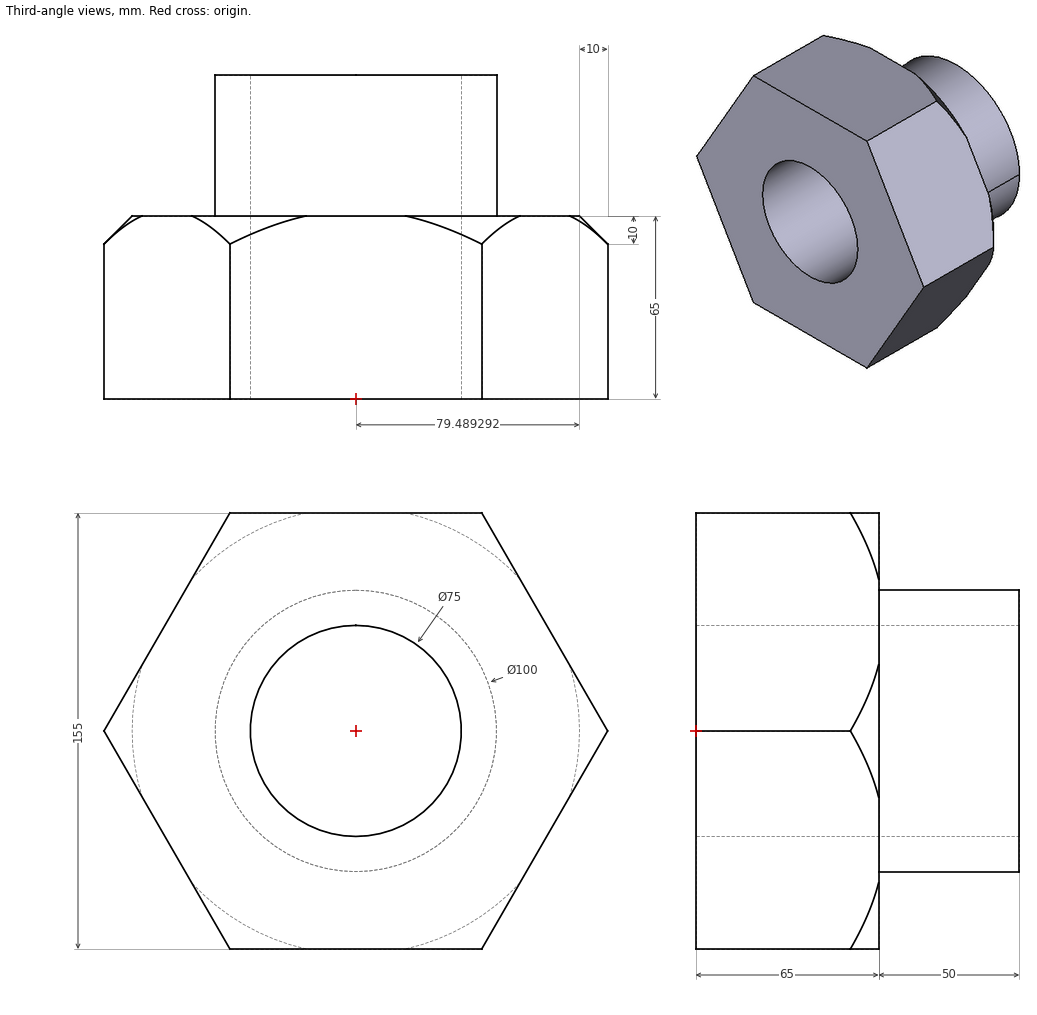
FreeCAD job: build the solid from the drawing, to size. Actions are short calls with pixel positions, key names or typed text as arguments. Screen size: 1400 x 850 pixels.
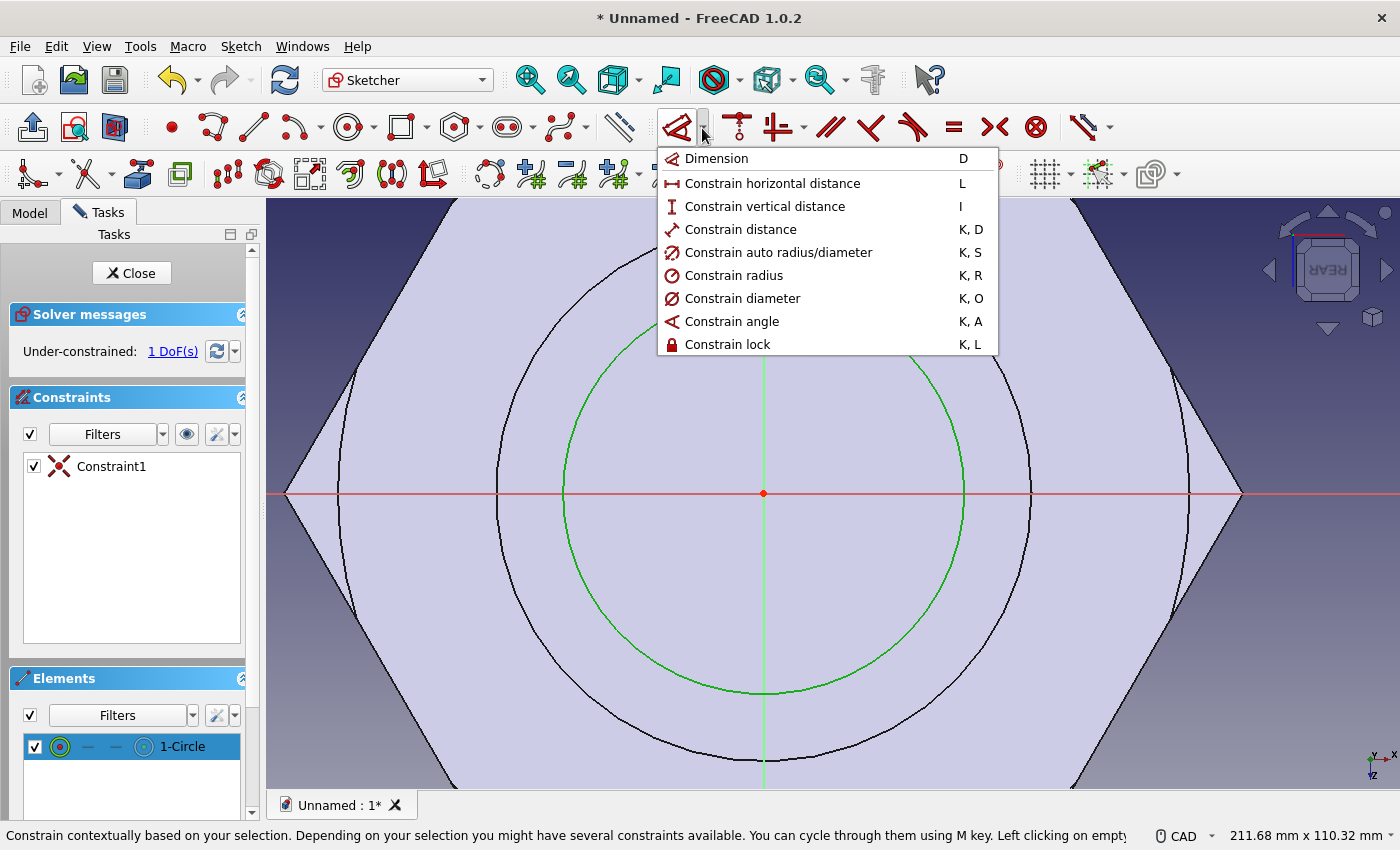
click(828, 298)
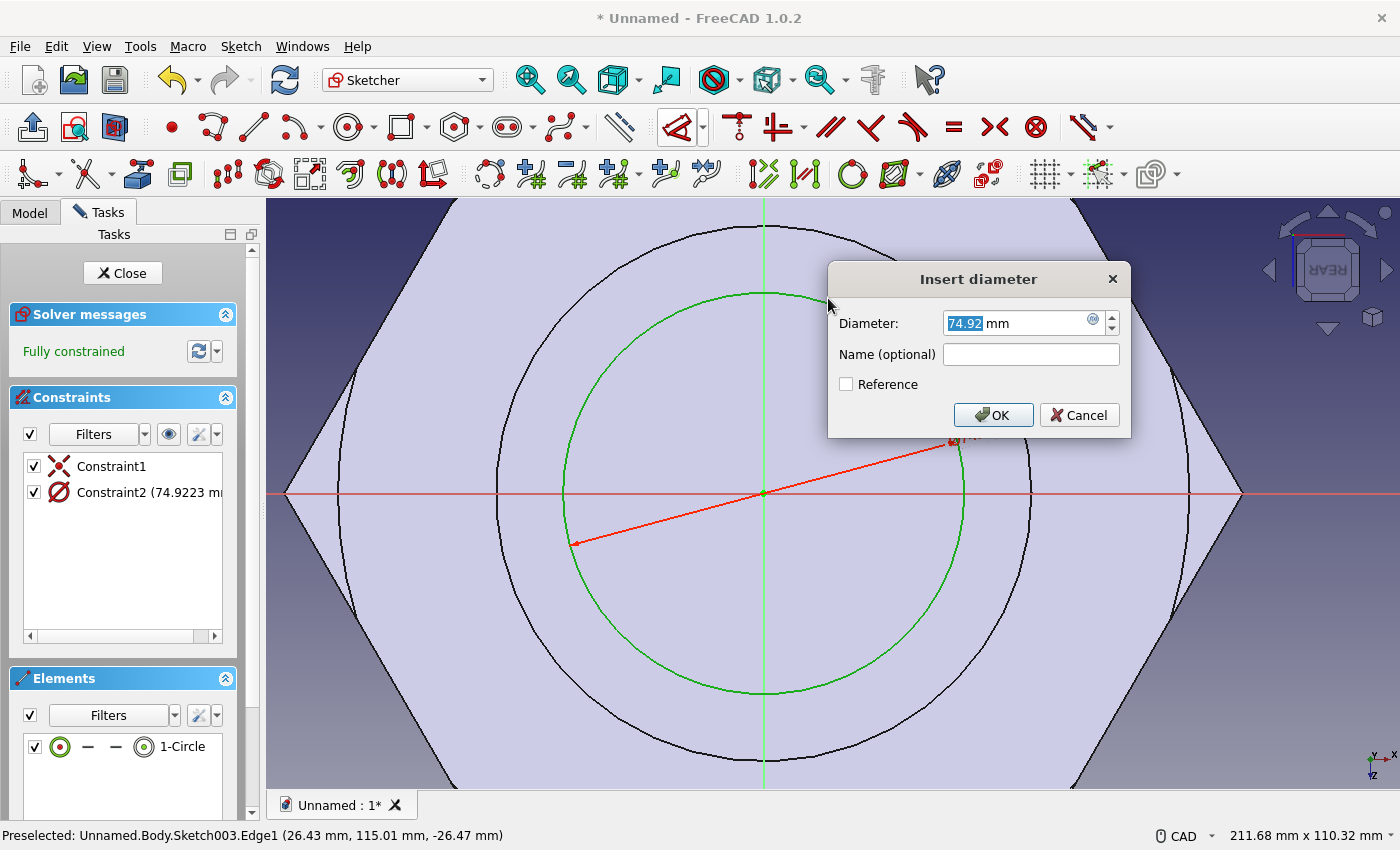
text(75)
key(Return)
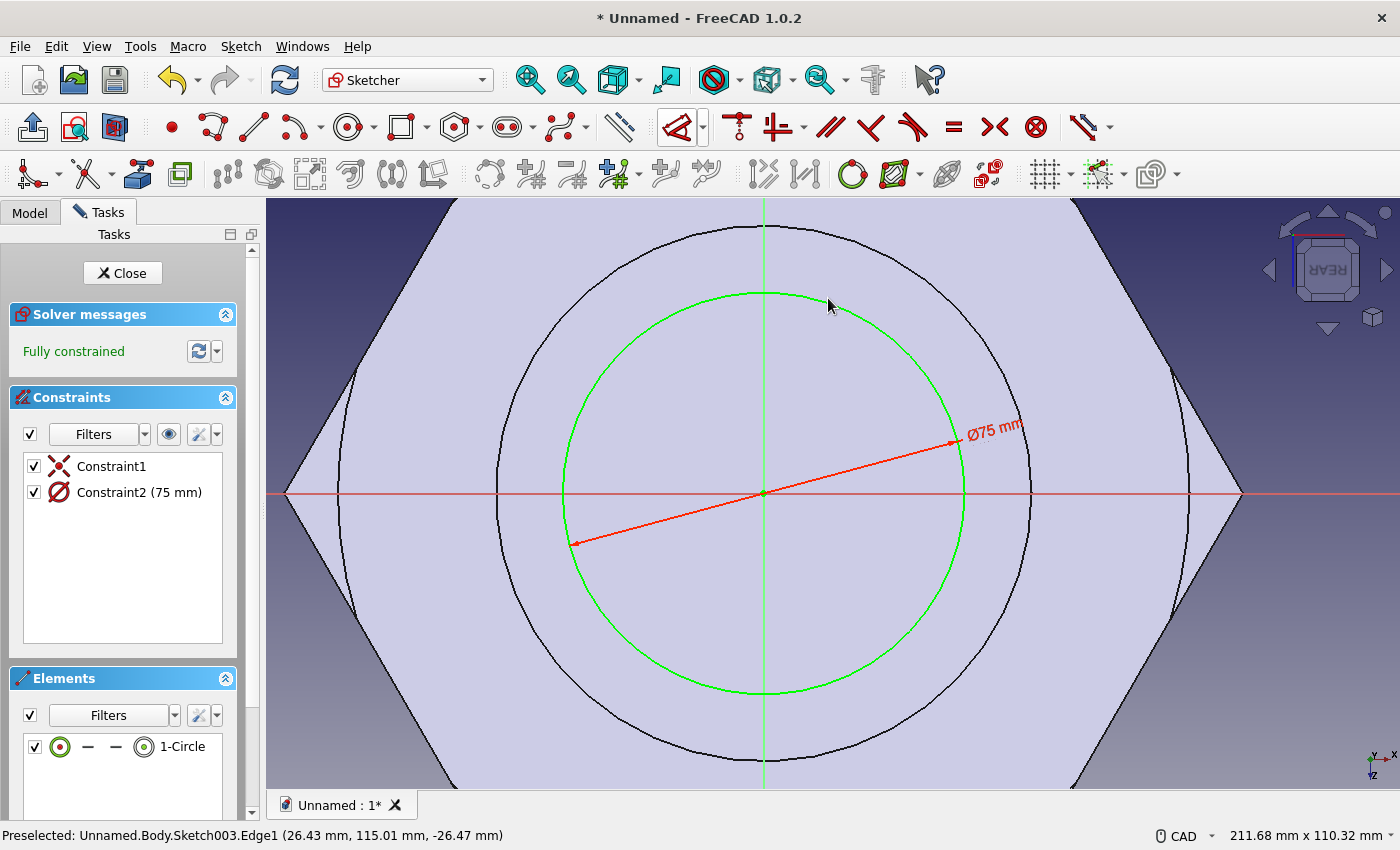
click(123, 273)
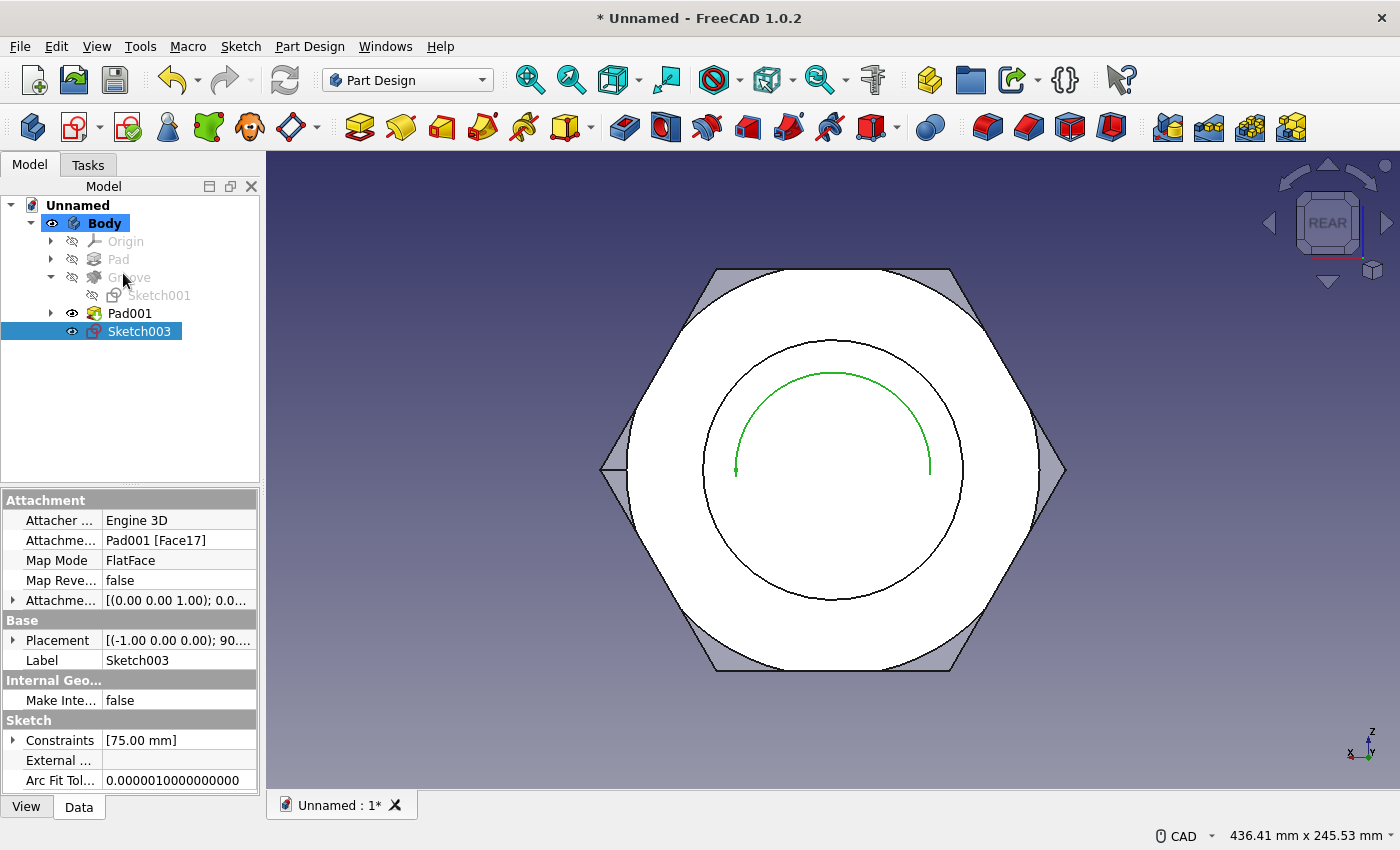
click(625, 128)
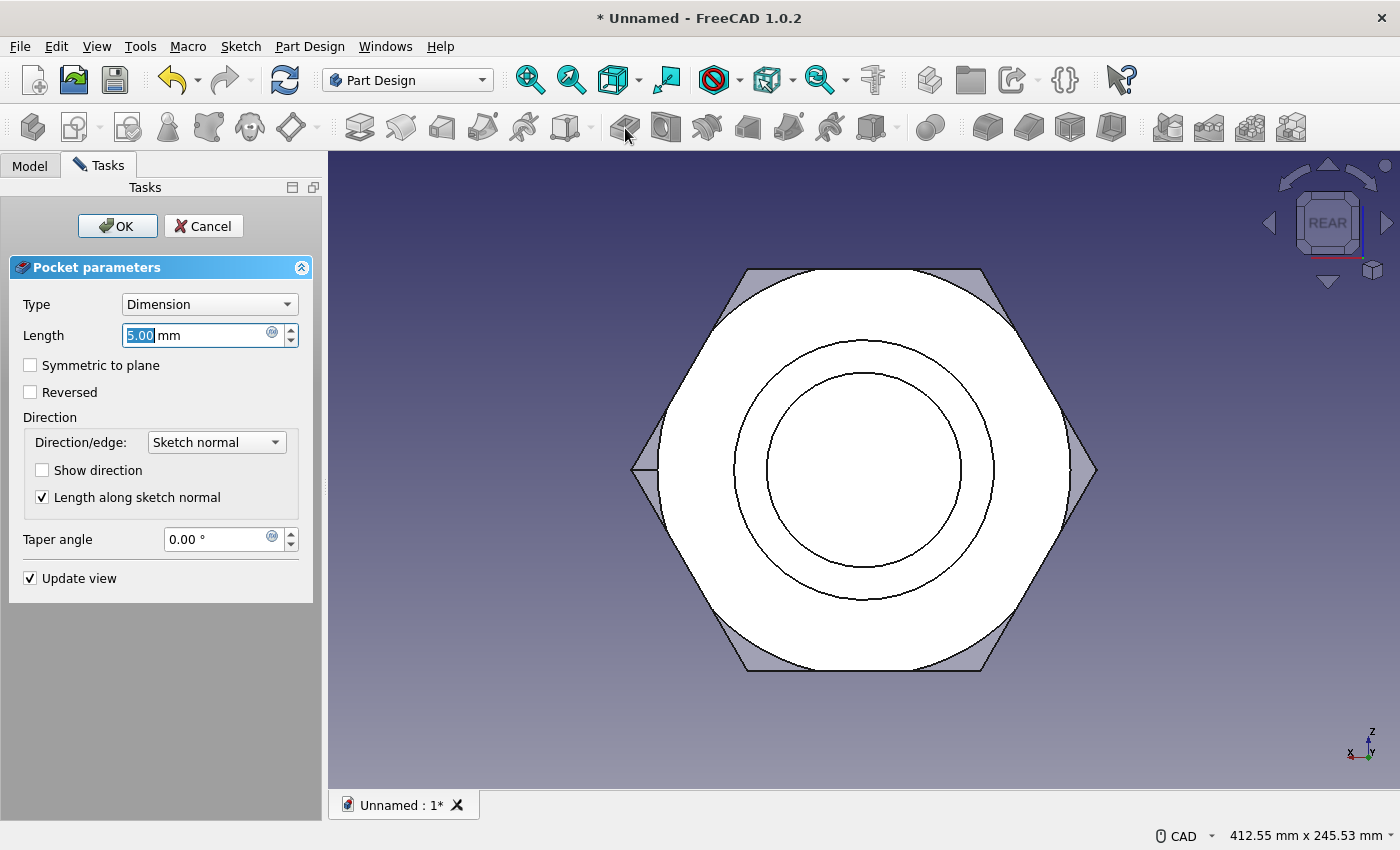
click(210, 304)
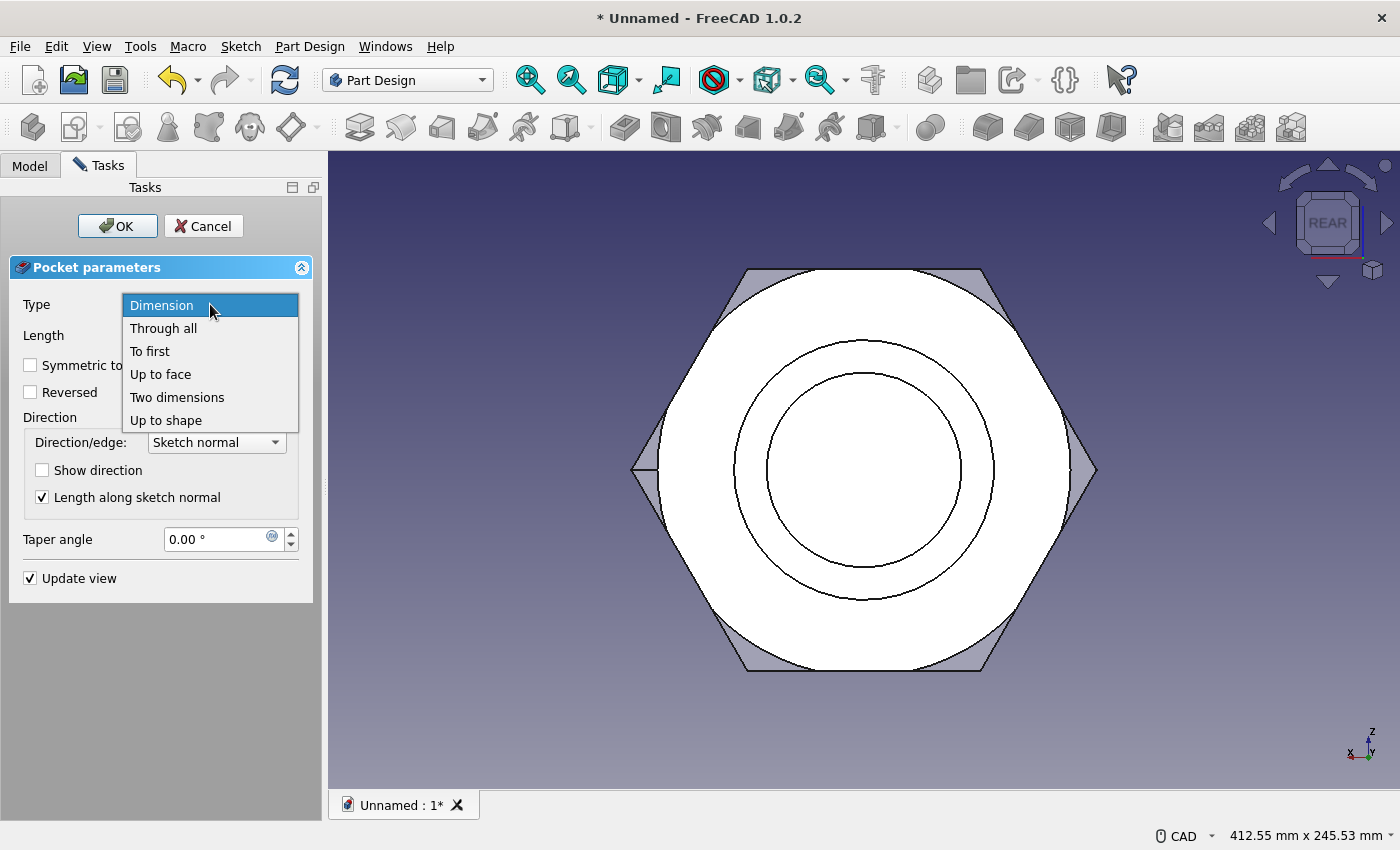
click(208, 352)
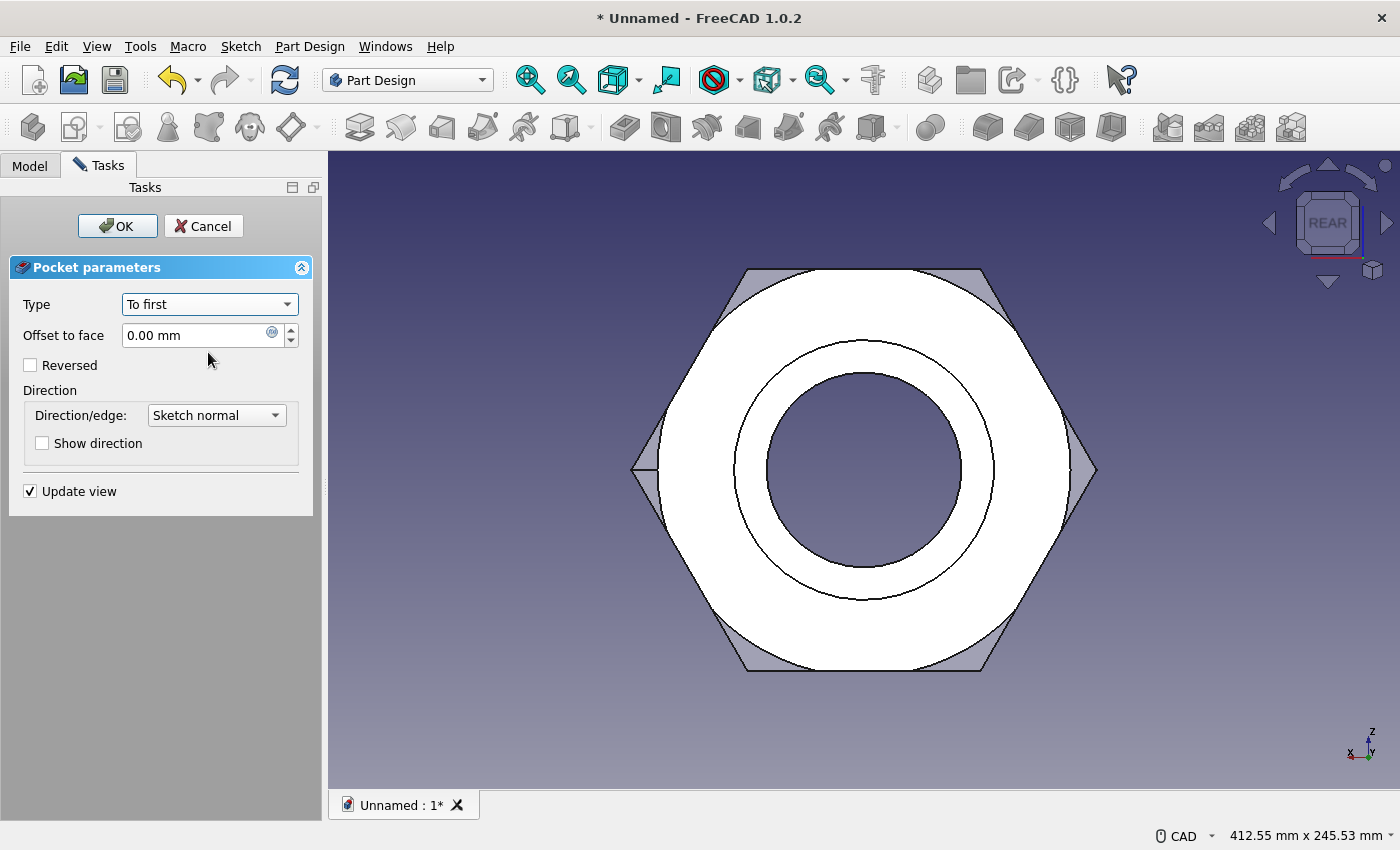
click(118, 226)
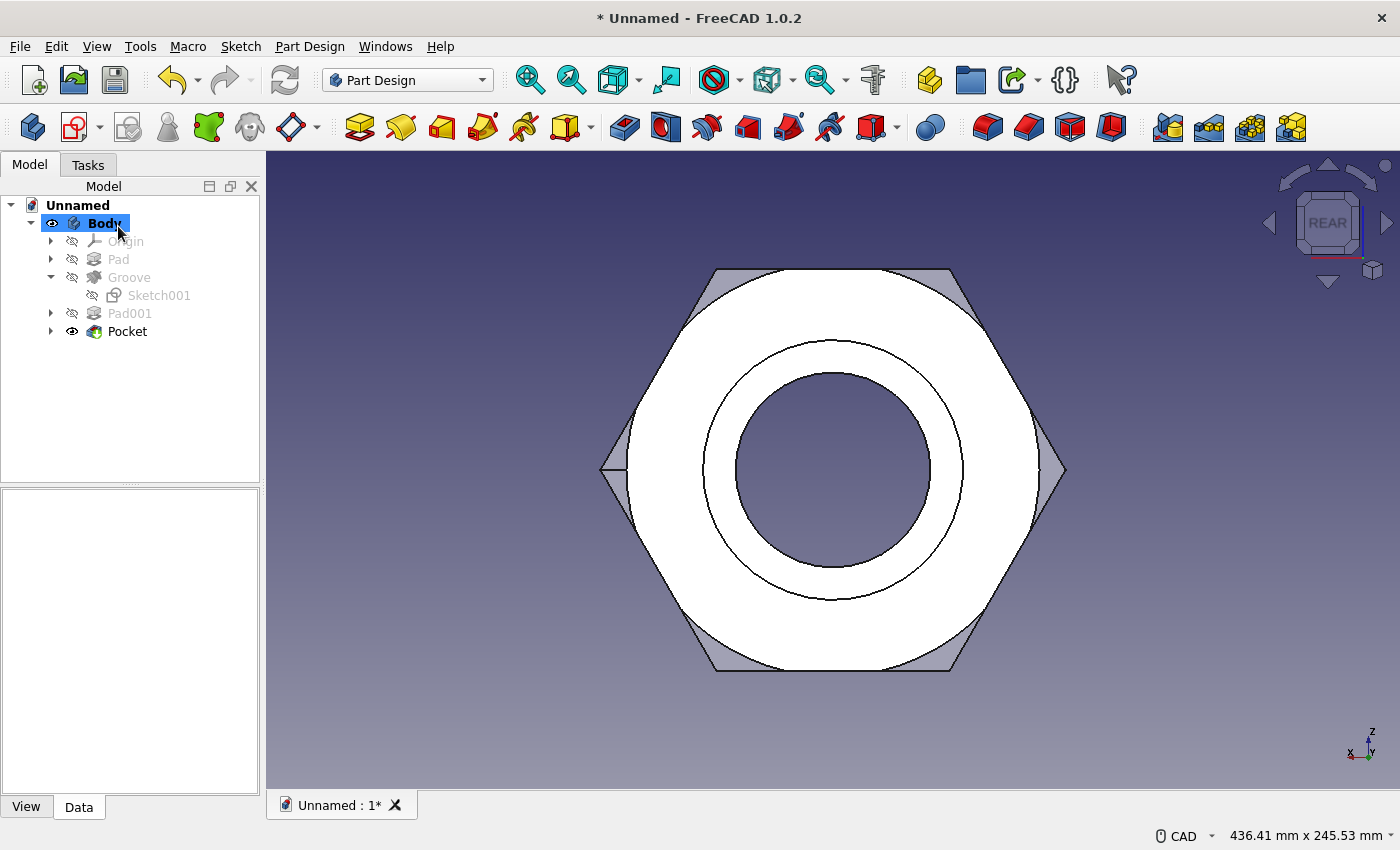
key(0)